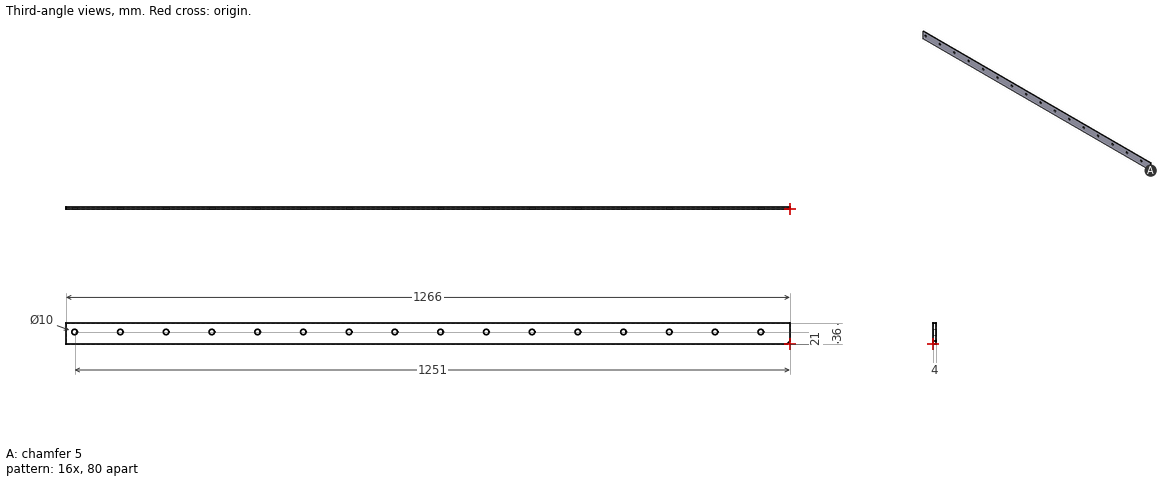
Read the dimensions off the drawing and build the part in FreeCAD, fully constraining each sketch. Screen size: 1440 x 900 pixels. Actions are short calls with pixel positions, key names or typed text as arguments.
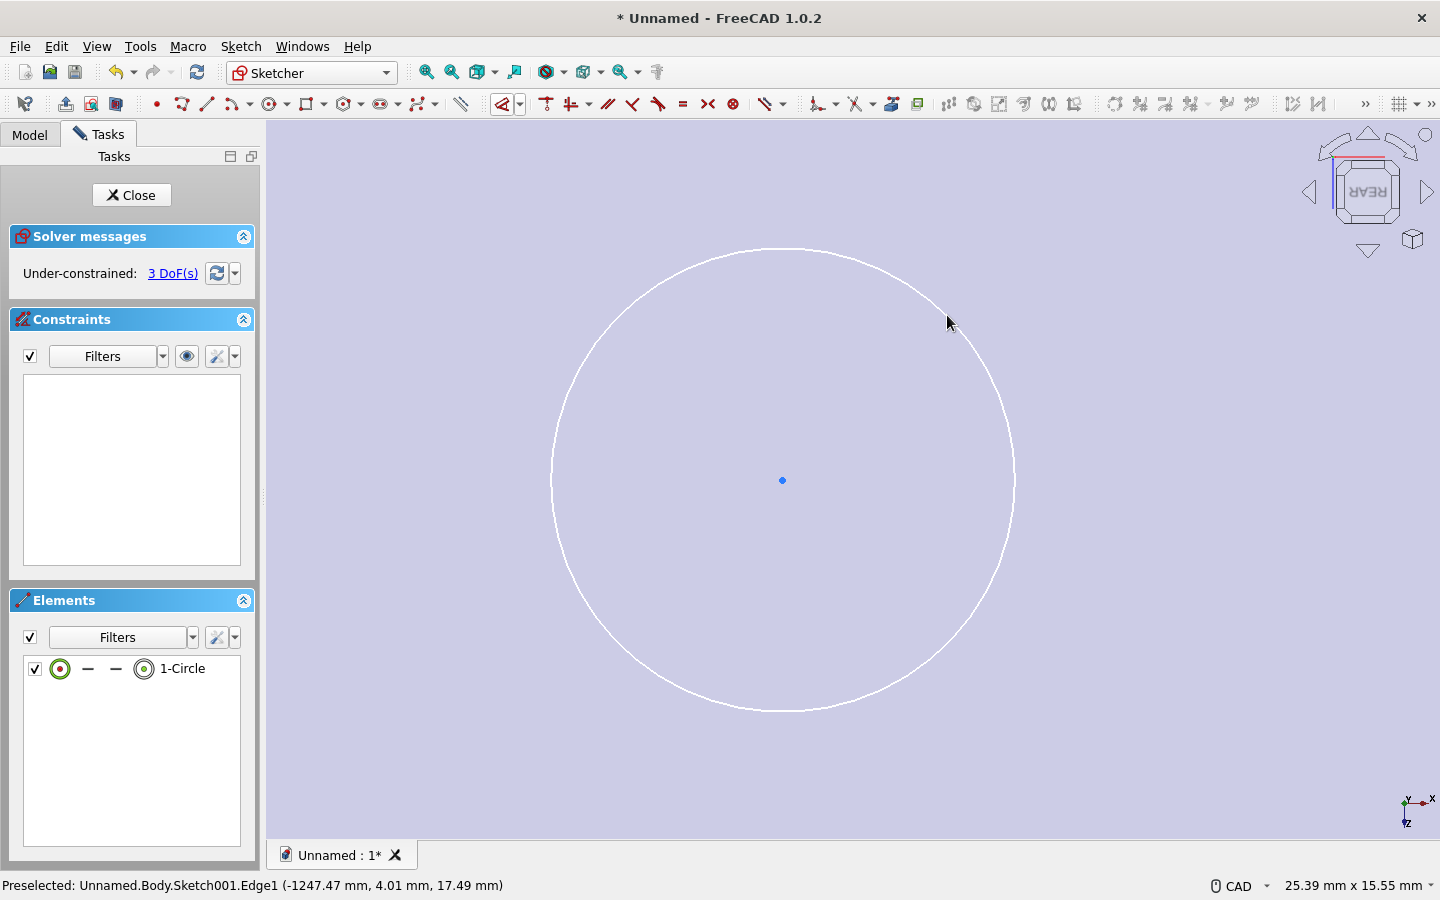
click(946, 315)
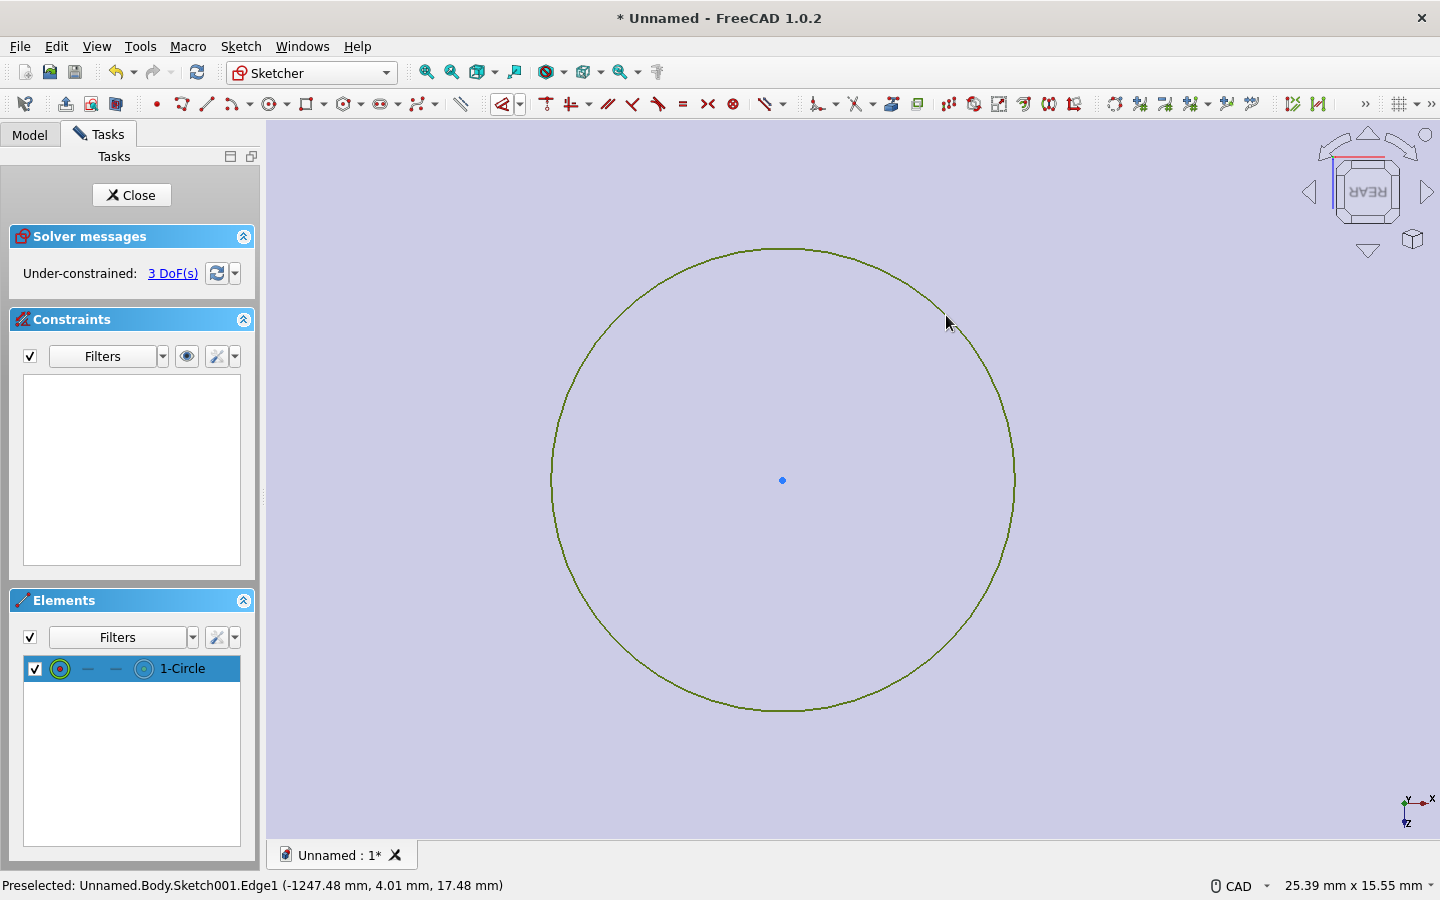
click(520, 104)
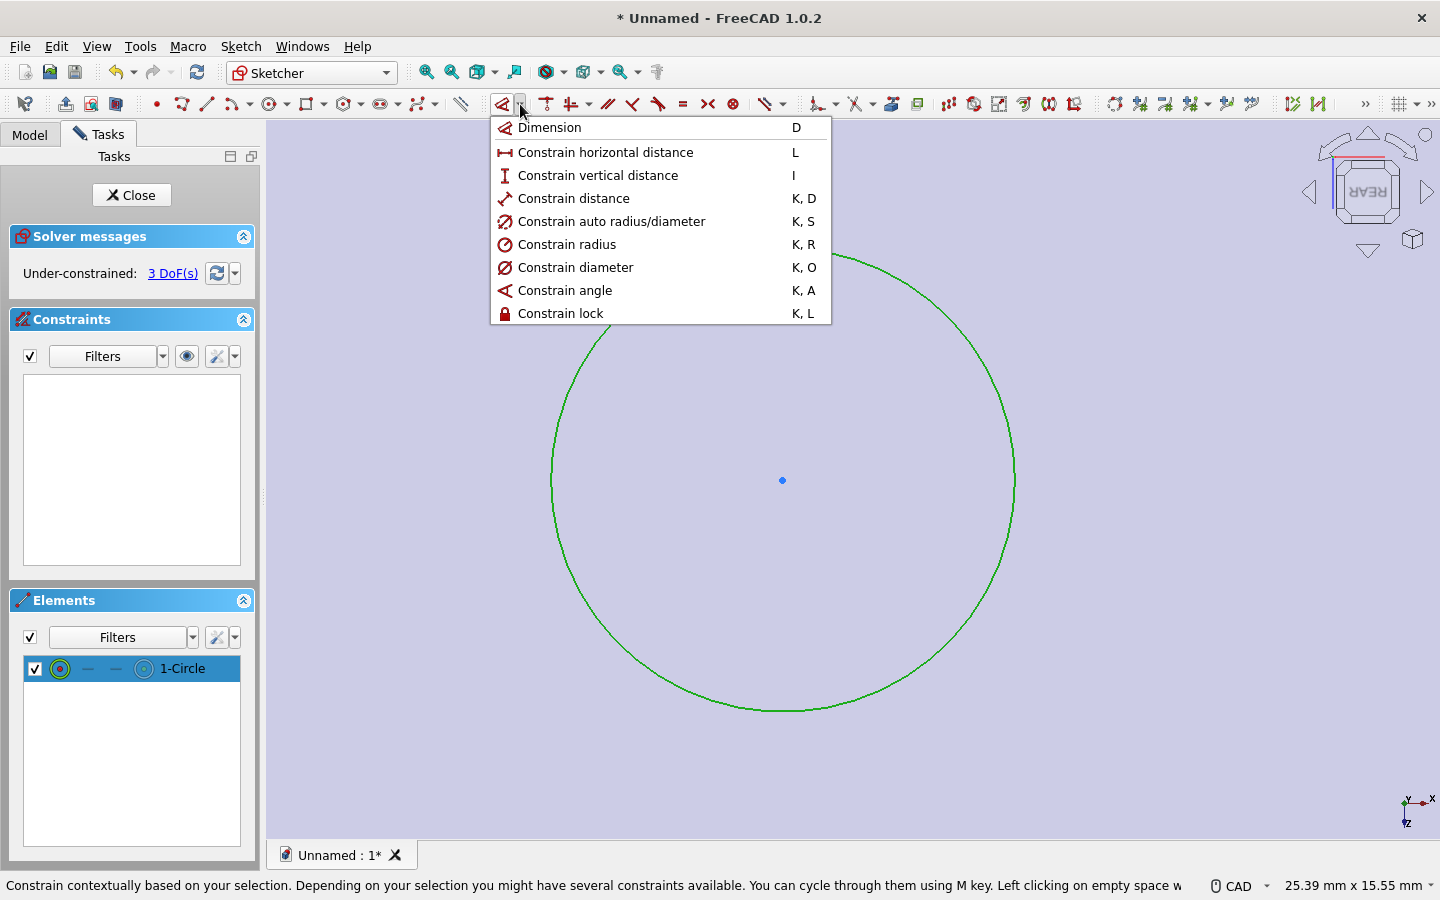
click(661, 268)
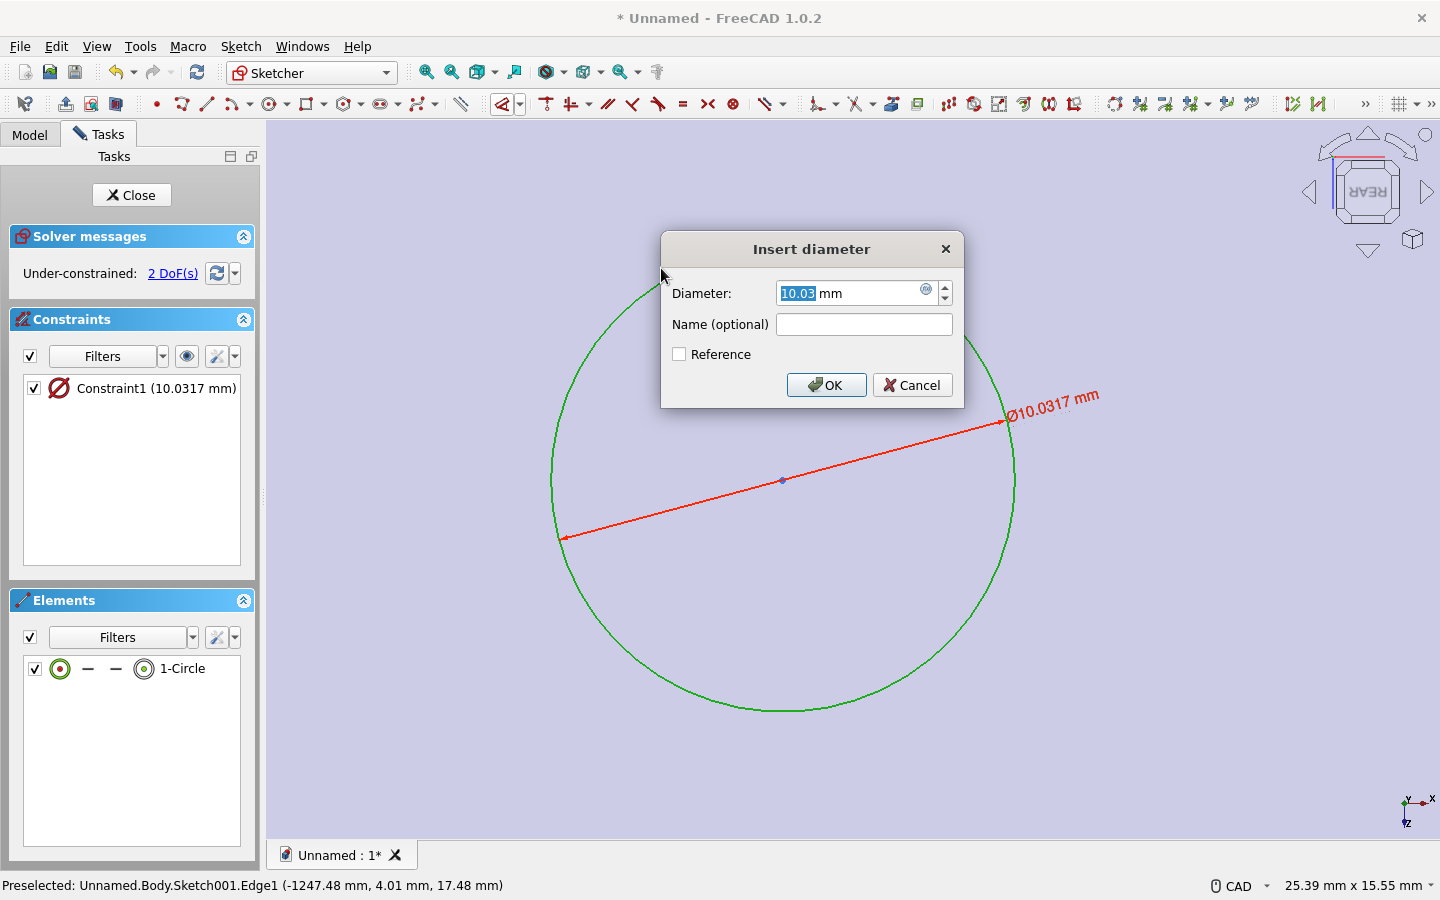
text(10)
key(Return)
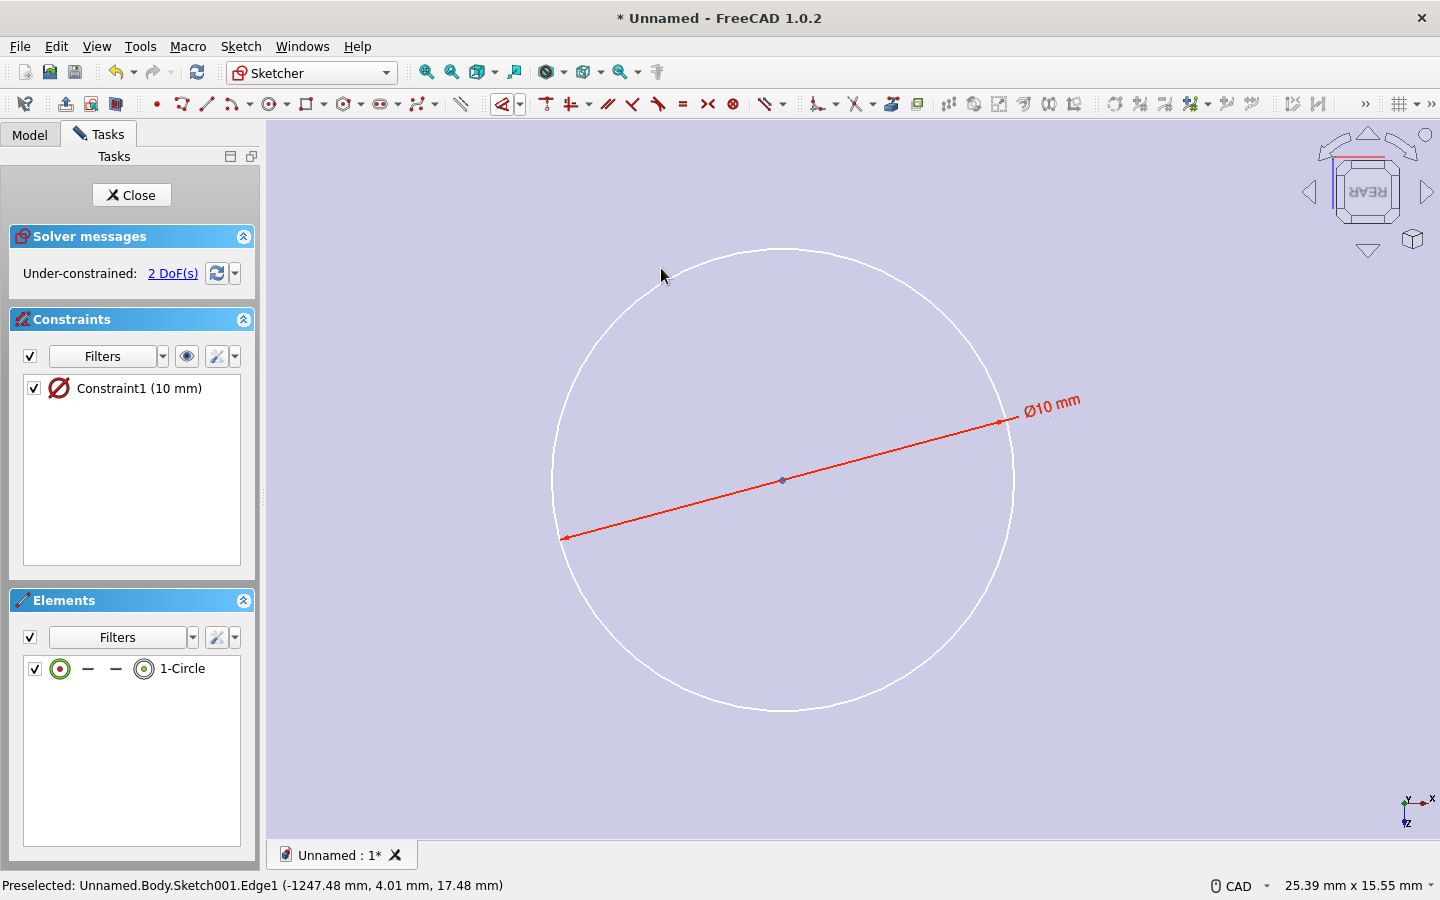
click(783, 480)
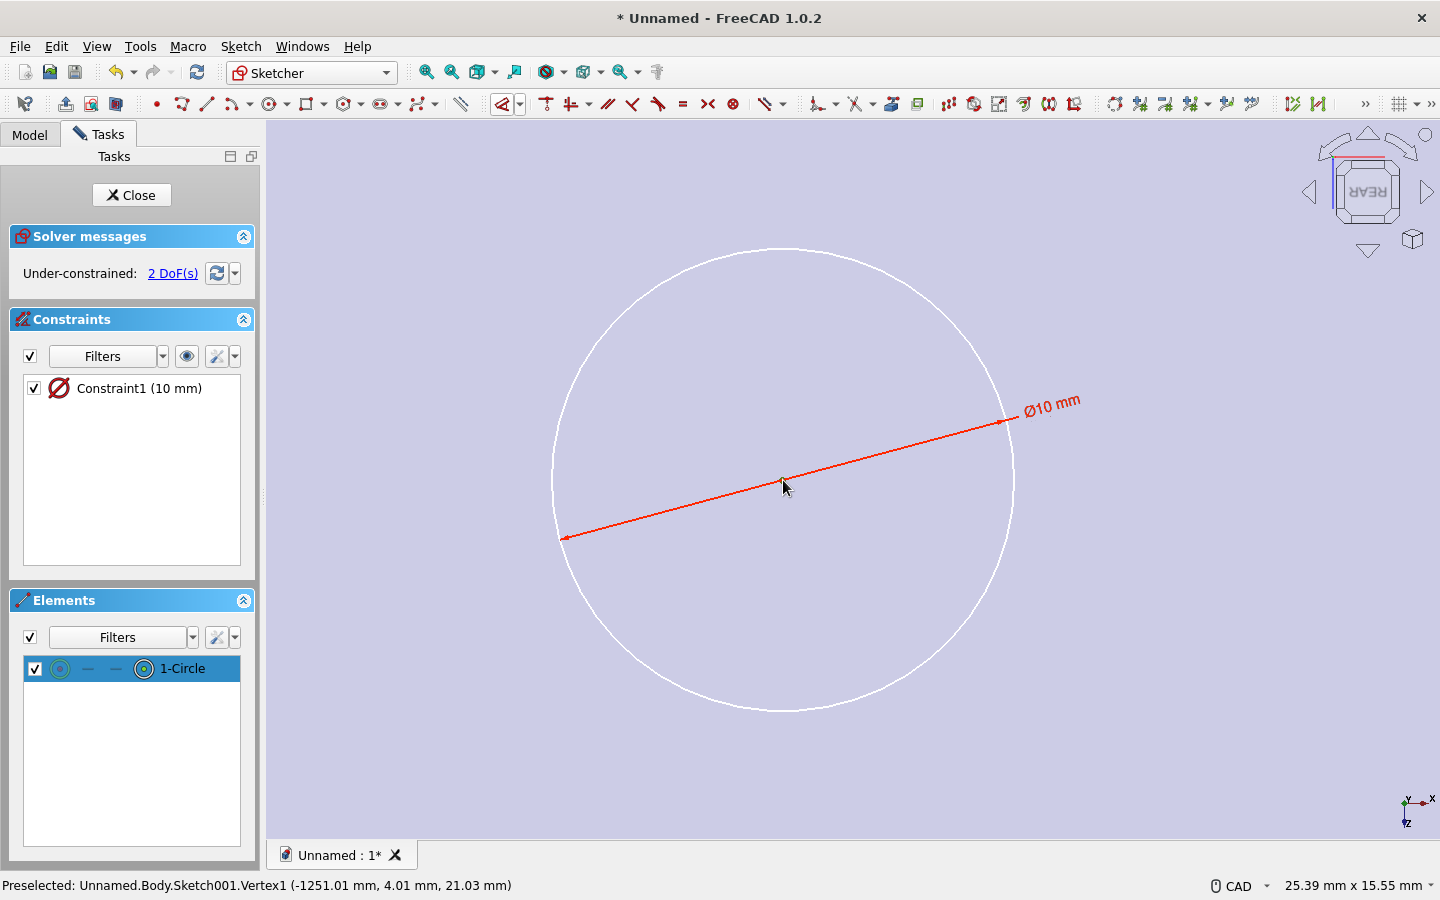
click(520, 104)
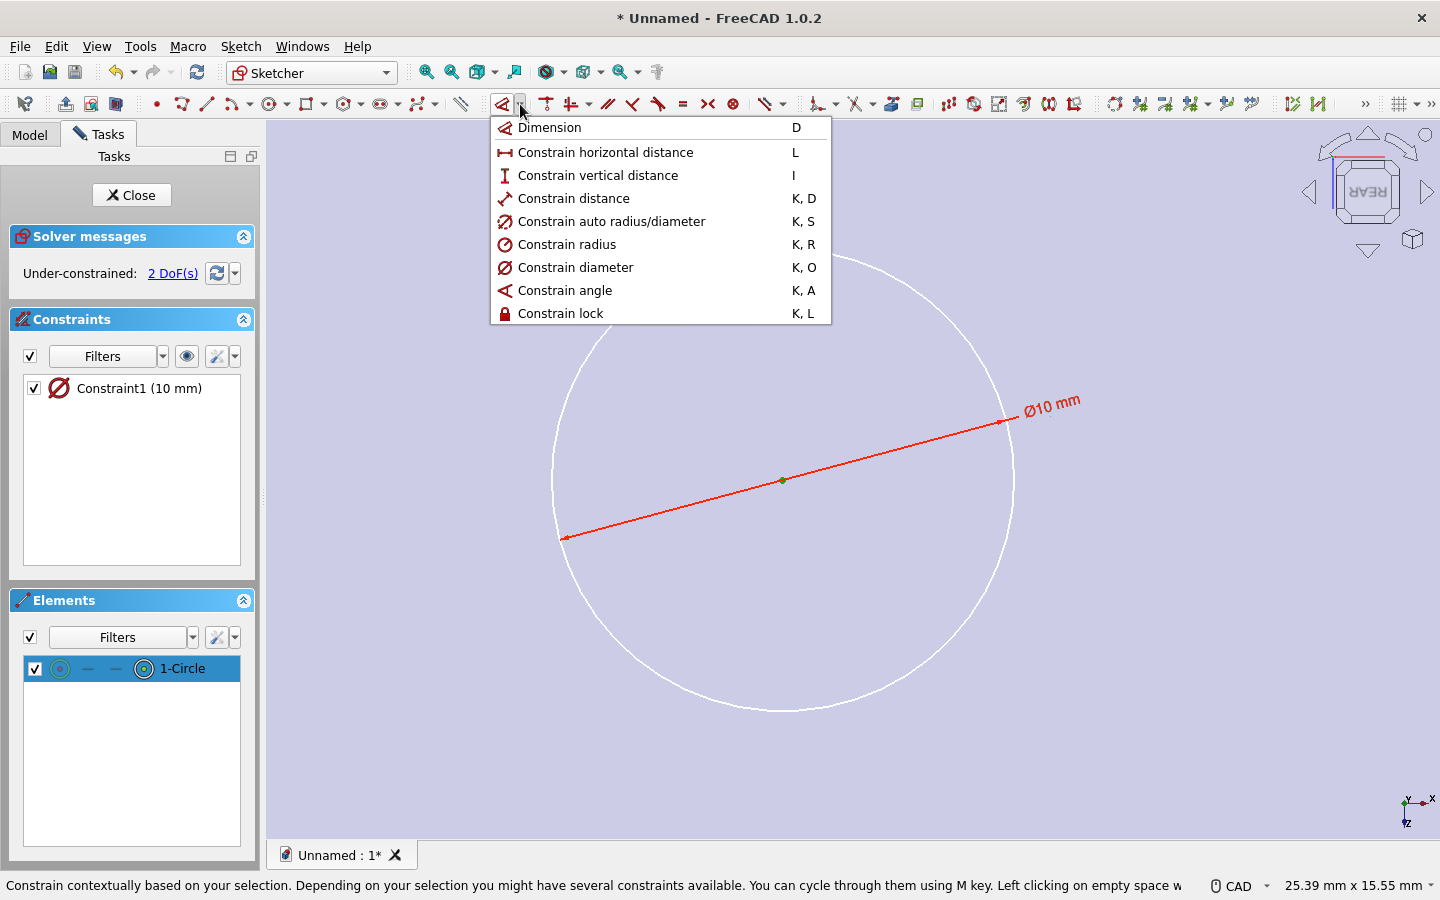
click(661, 176)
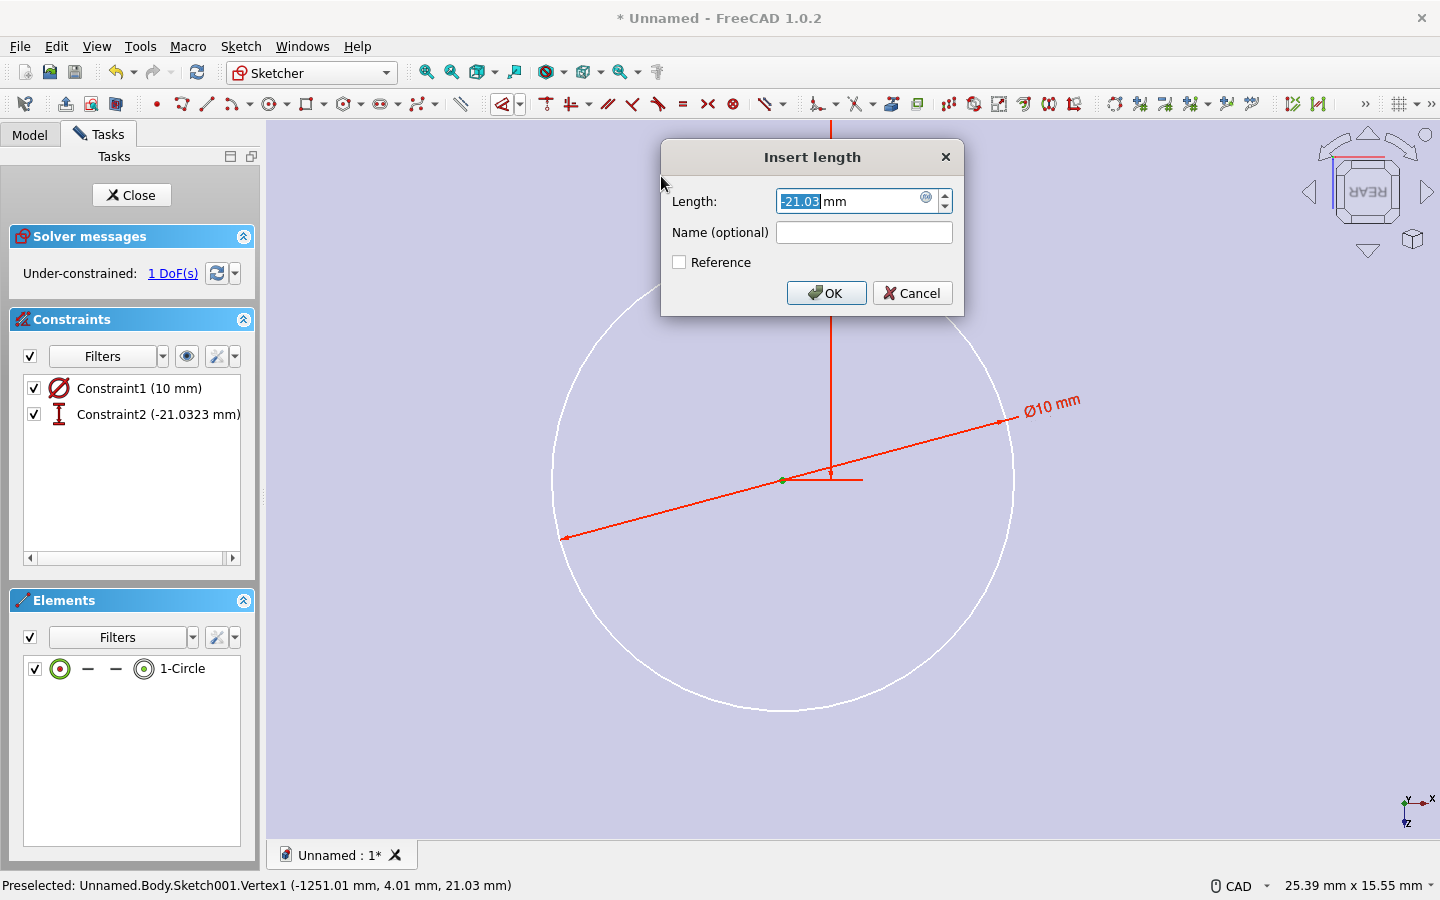
text(-21)
key(Return)